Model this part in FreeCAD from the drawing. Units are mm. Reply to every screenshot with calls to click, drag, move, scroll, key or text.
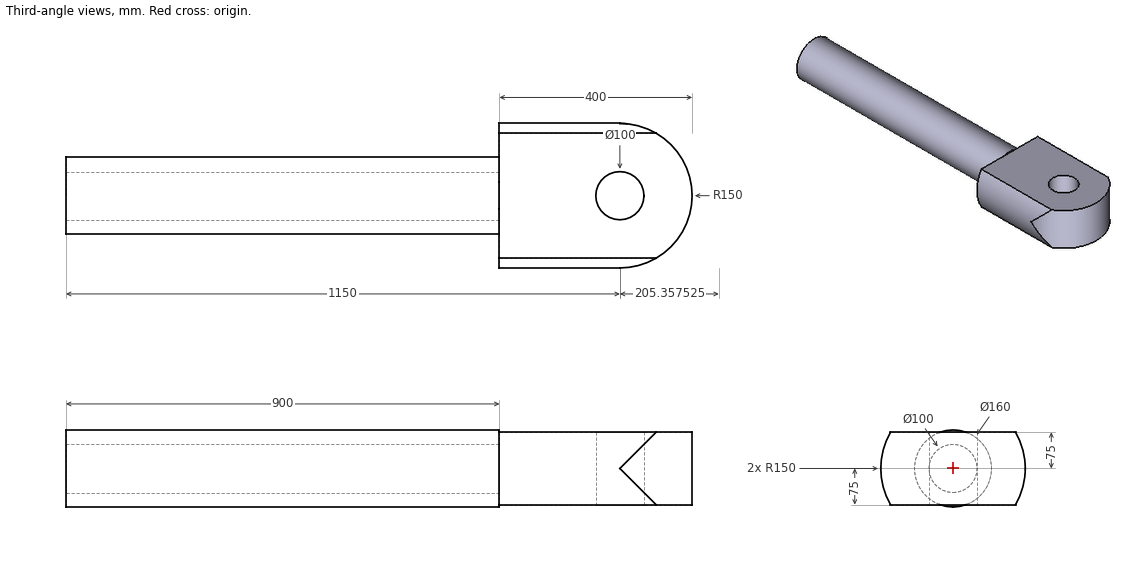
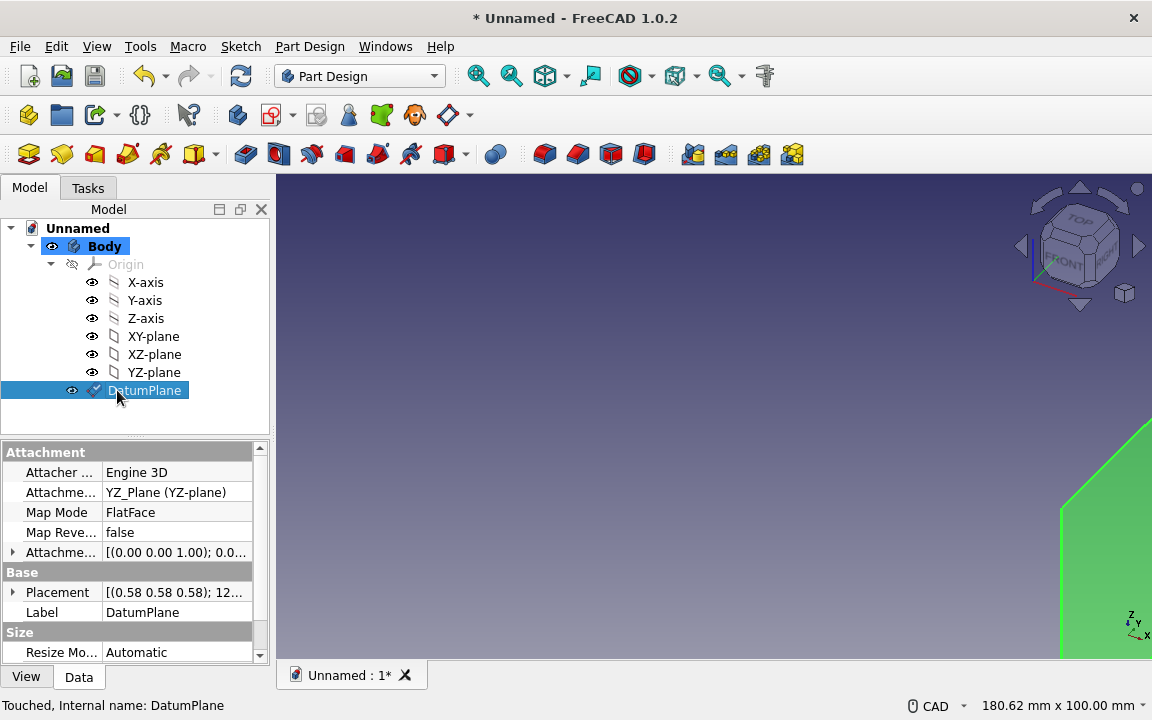
click(270, 116)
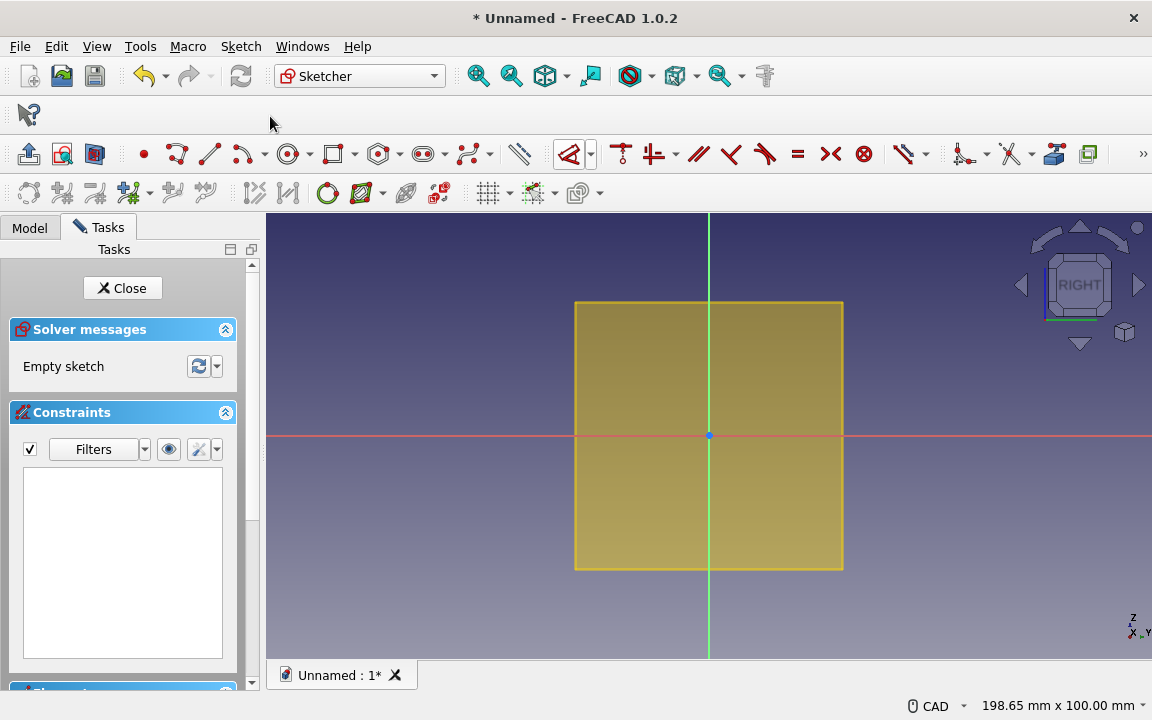
scroll(601, 436, down, 5)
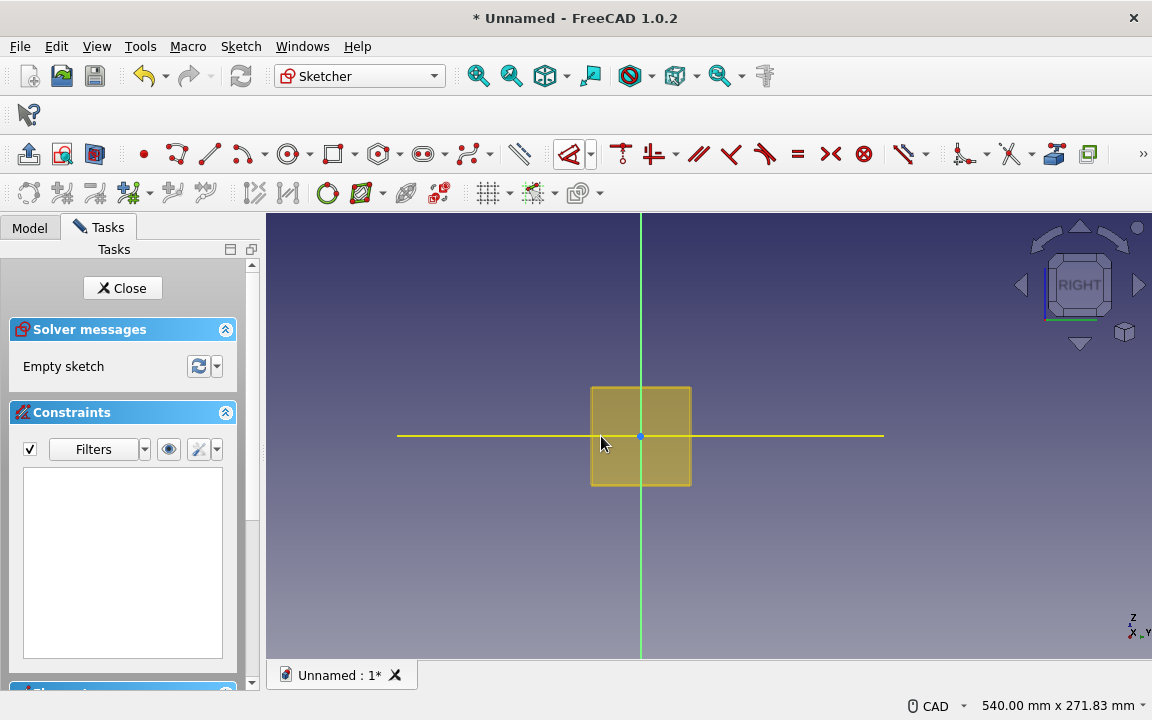
click(288, 154)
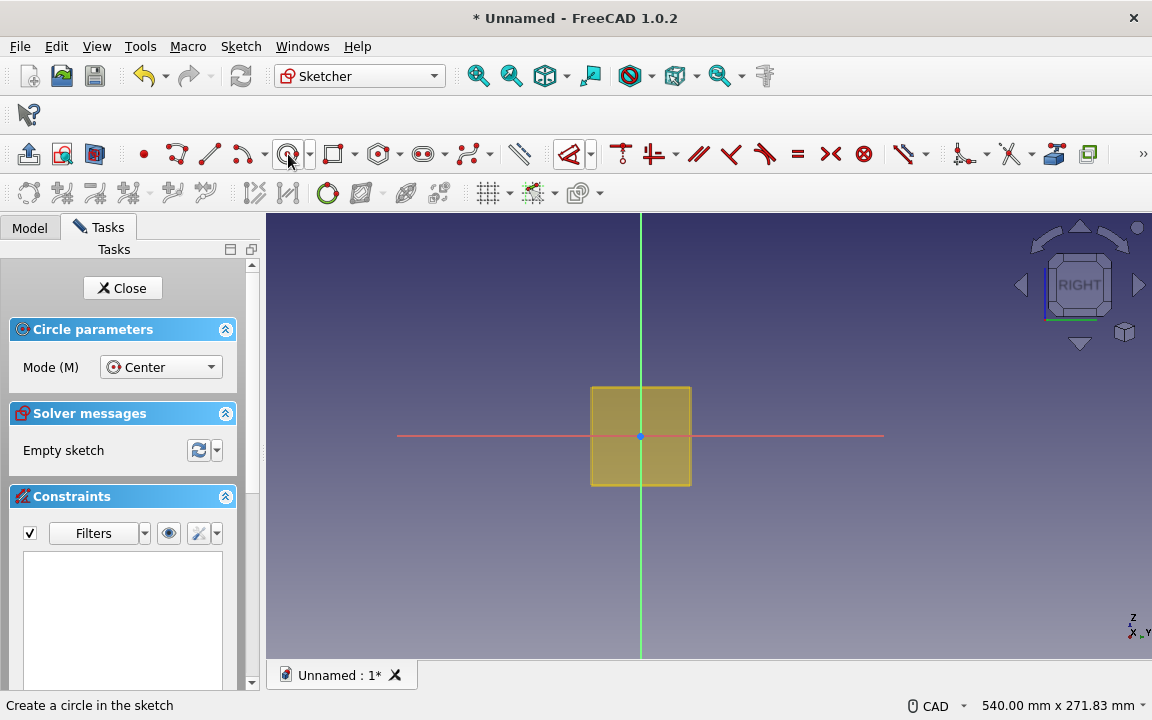
click(641, 436)
move(734, 344)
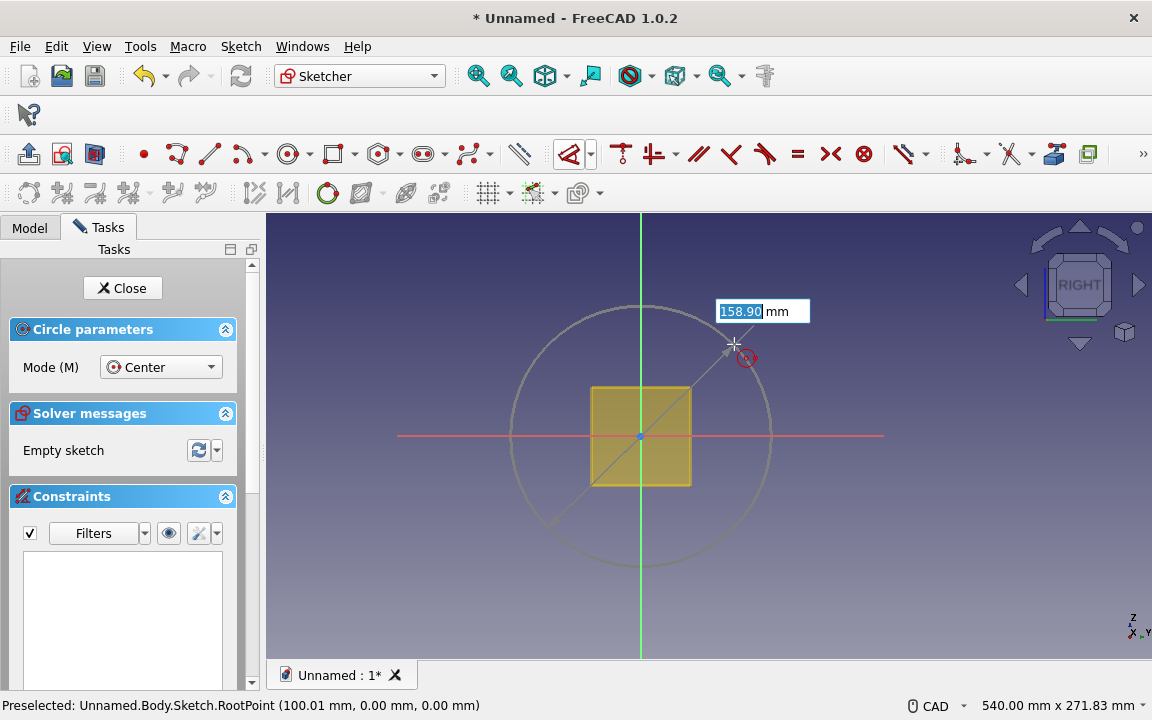
text(160)
key(Return)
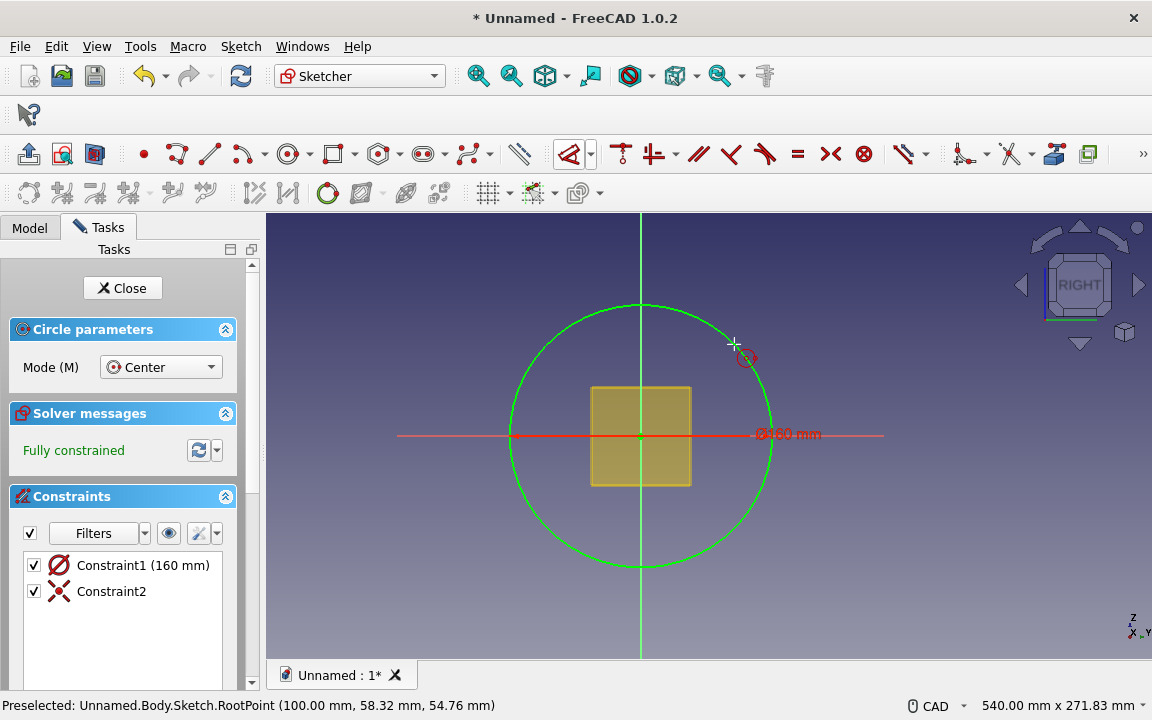
click(641, 436)
move(699, 378)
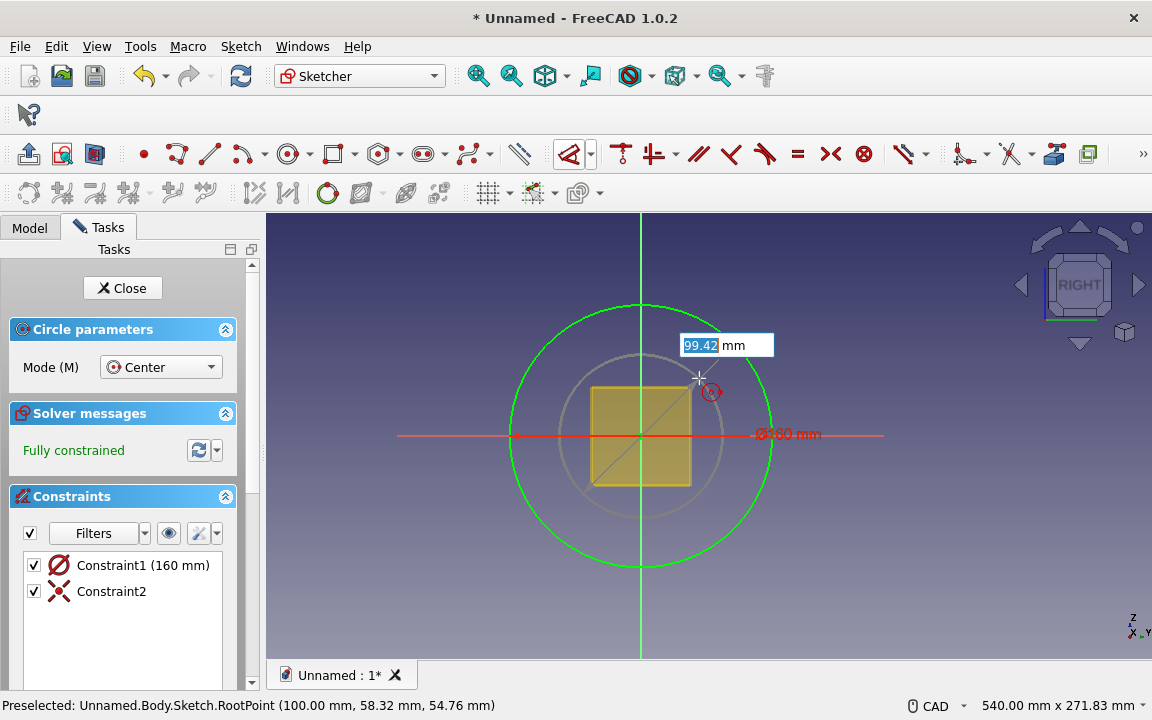
text(100)
key(Return)
key(Escape)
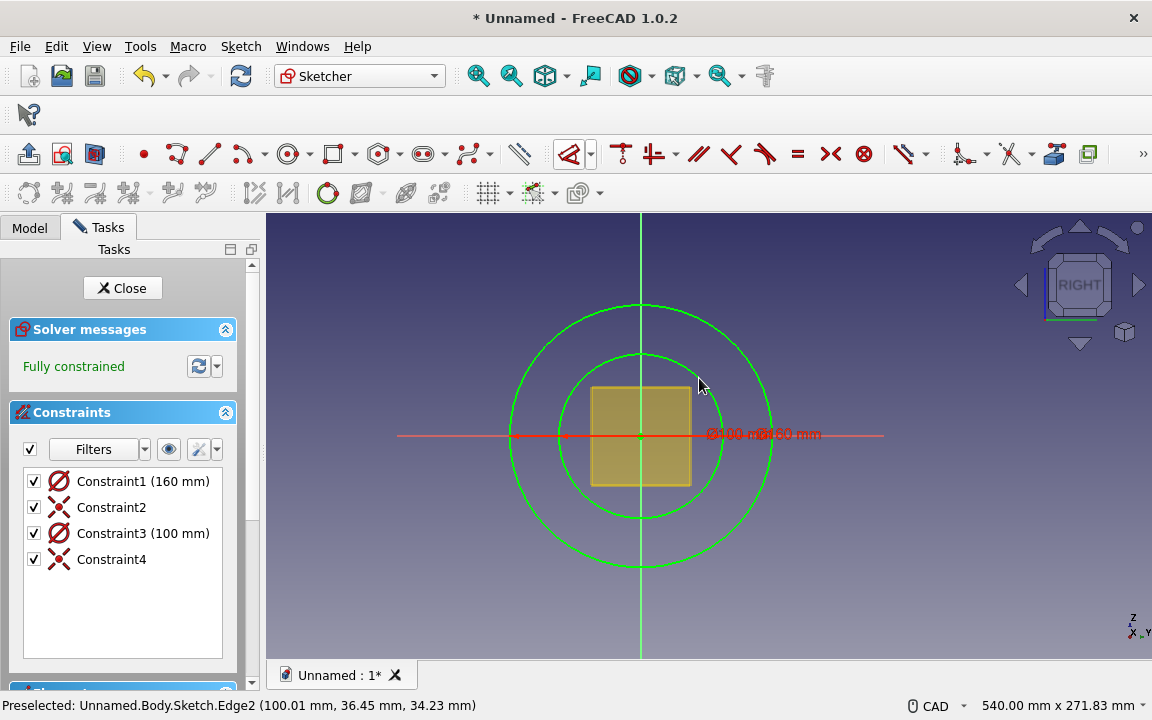
click(123, 288)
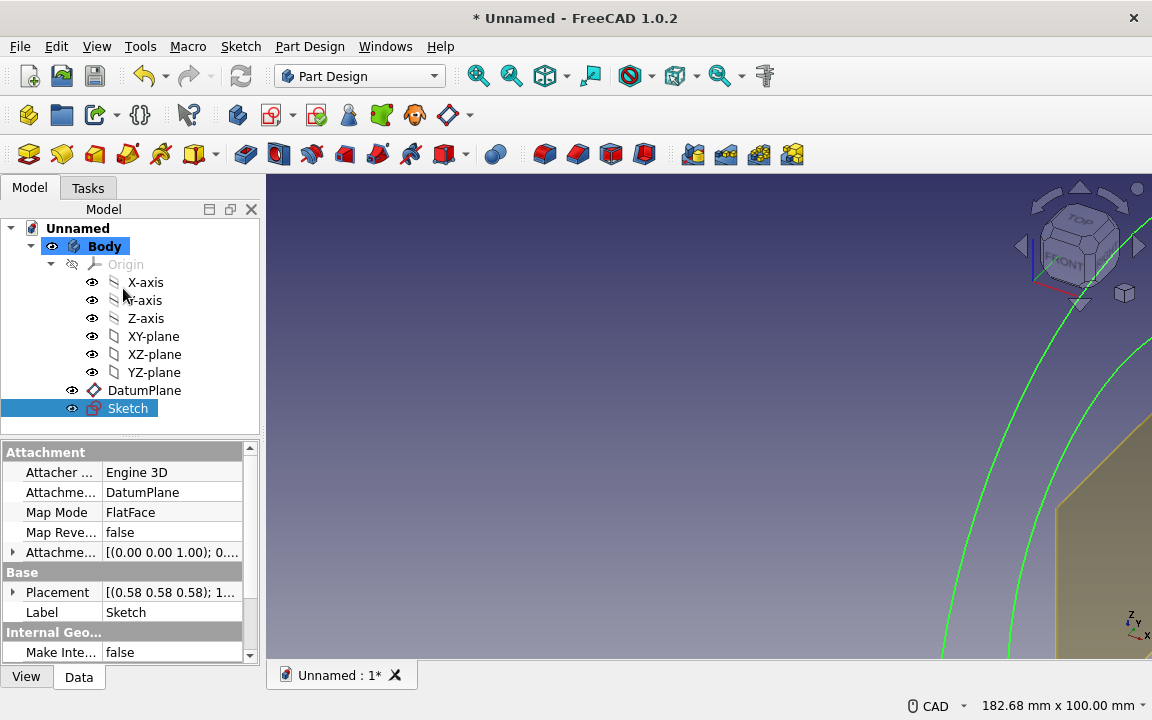
click(29, 154)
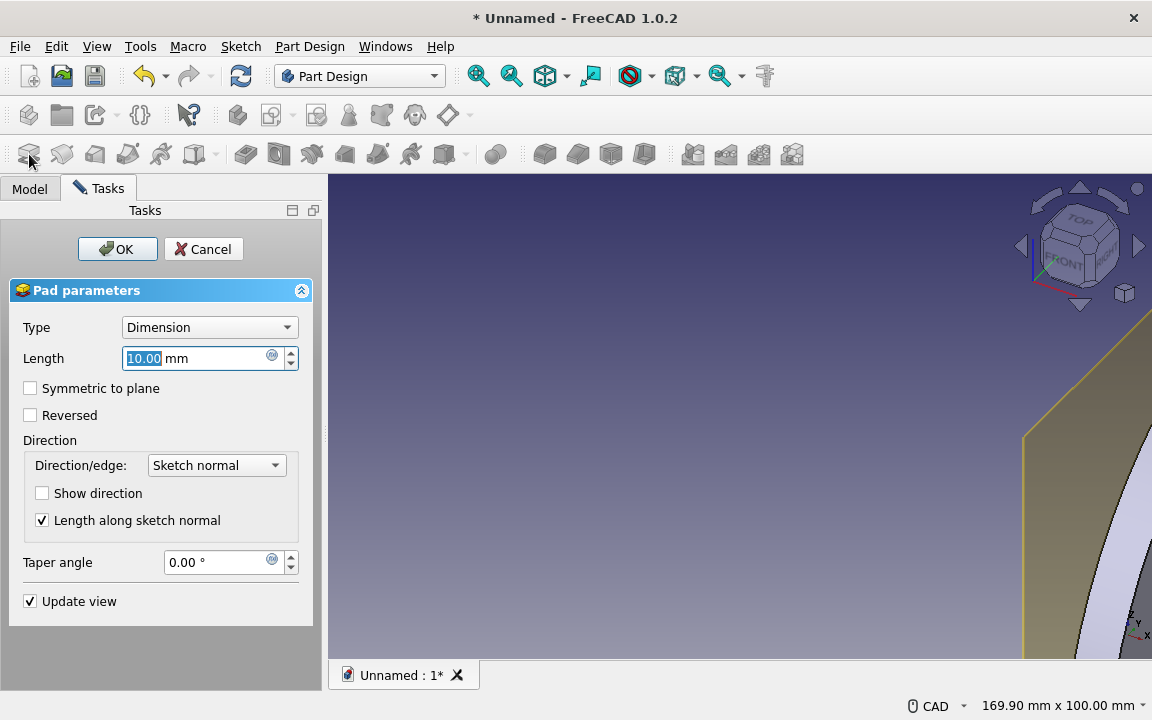
text(900)
key(Tab)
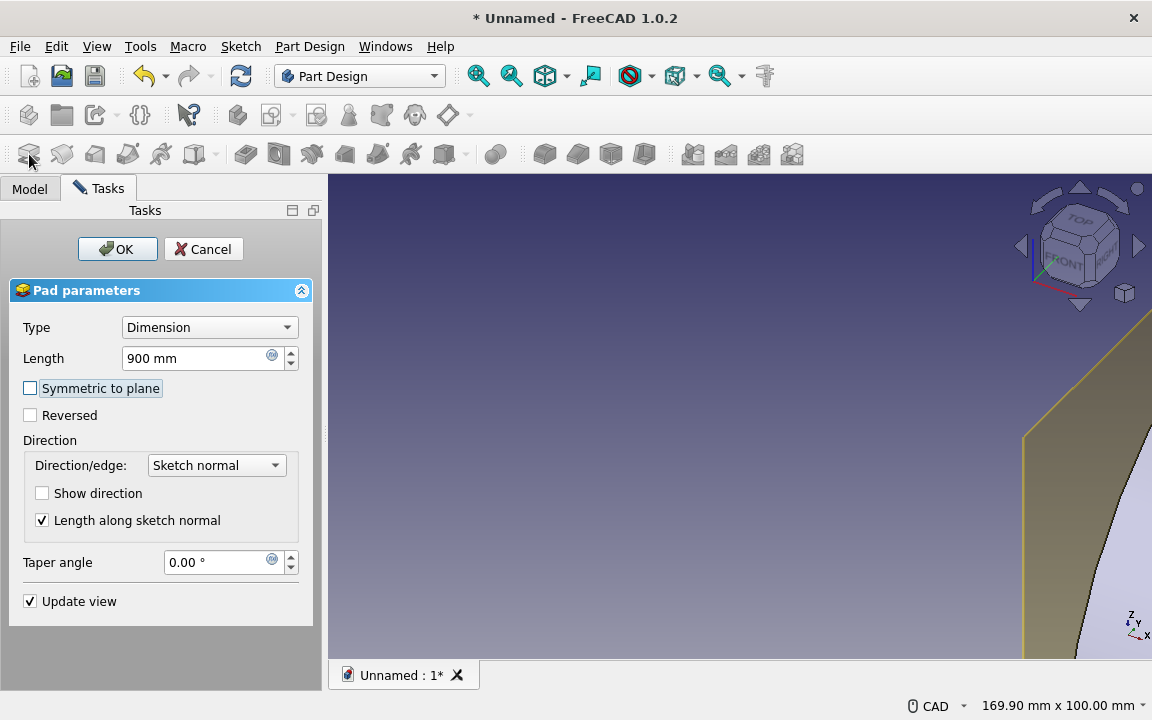
click(118, 249)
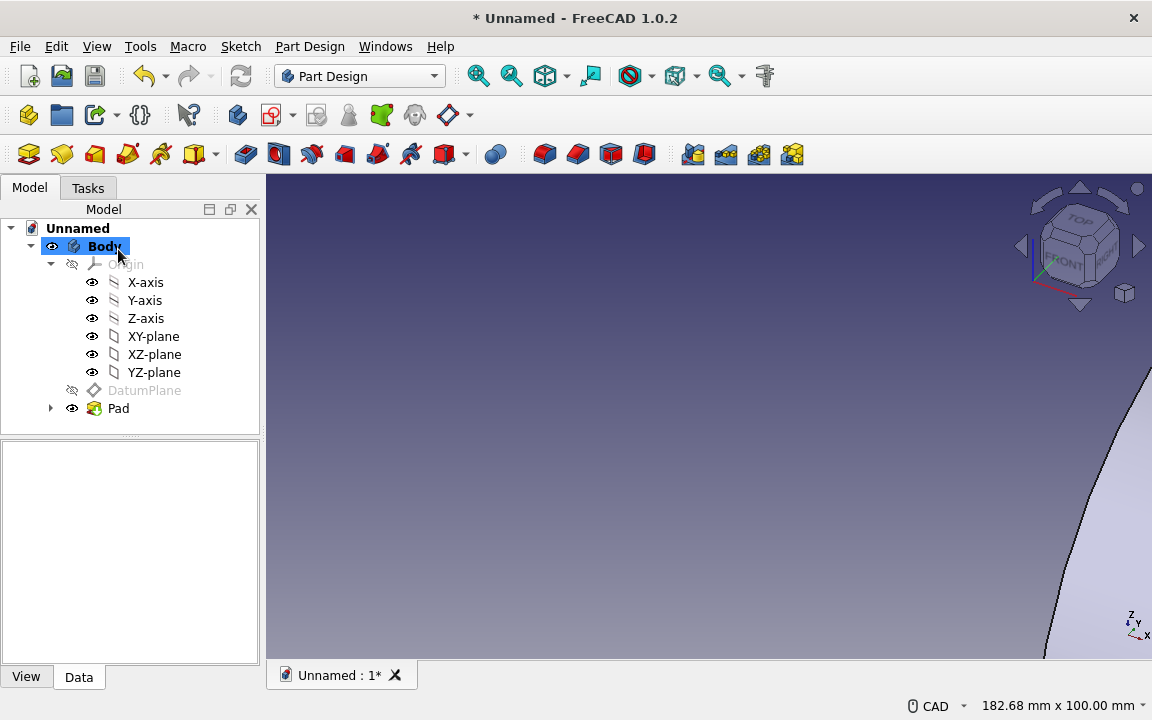
key(v)
key(f)